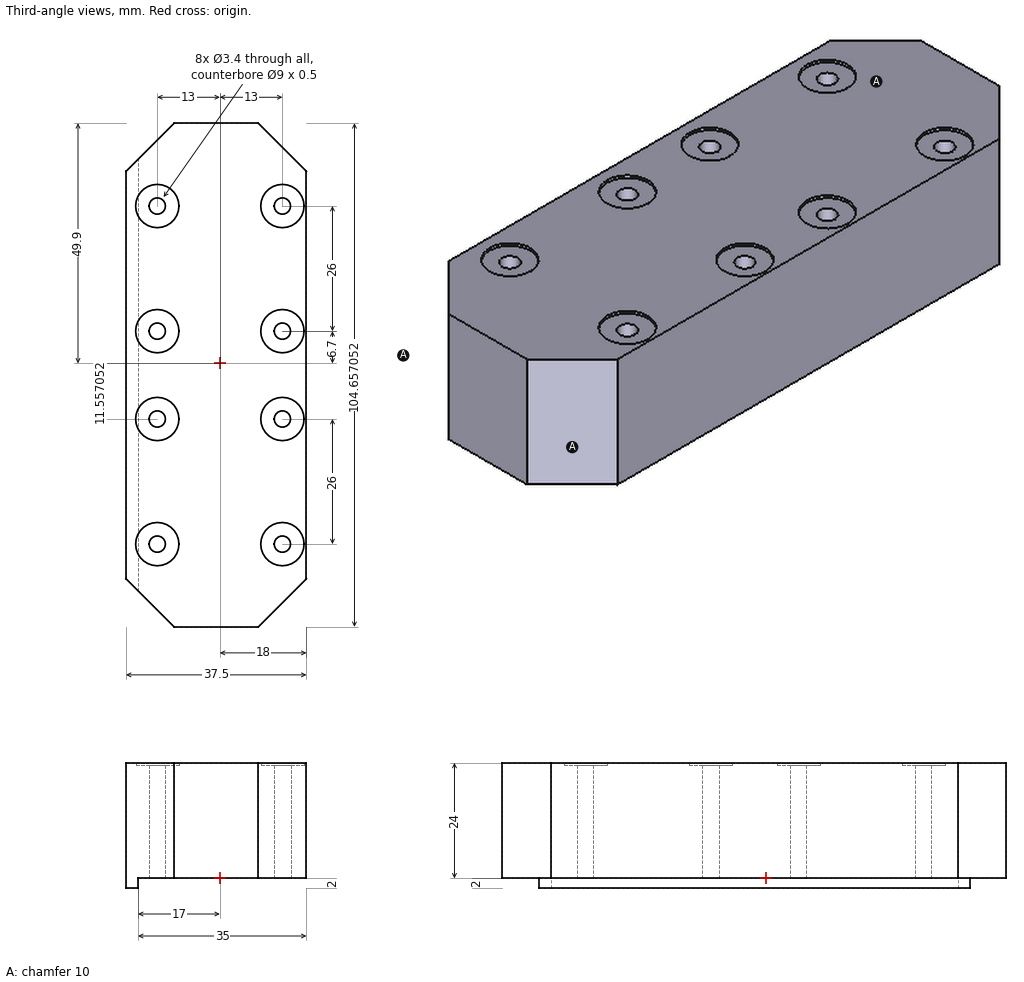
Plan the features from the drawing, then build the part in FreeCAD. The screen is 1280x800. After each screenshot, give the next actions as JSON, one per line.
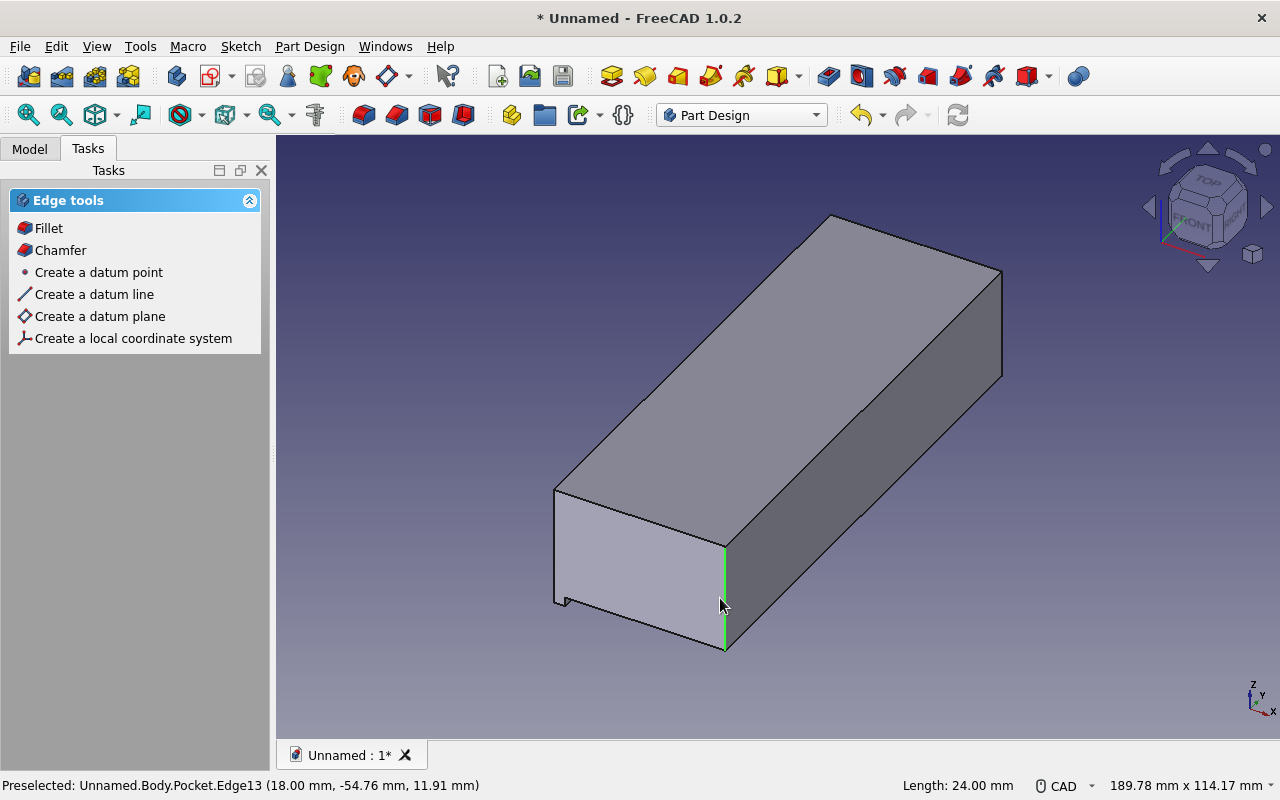
{"action": "key", "text": "0"}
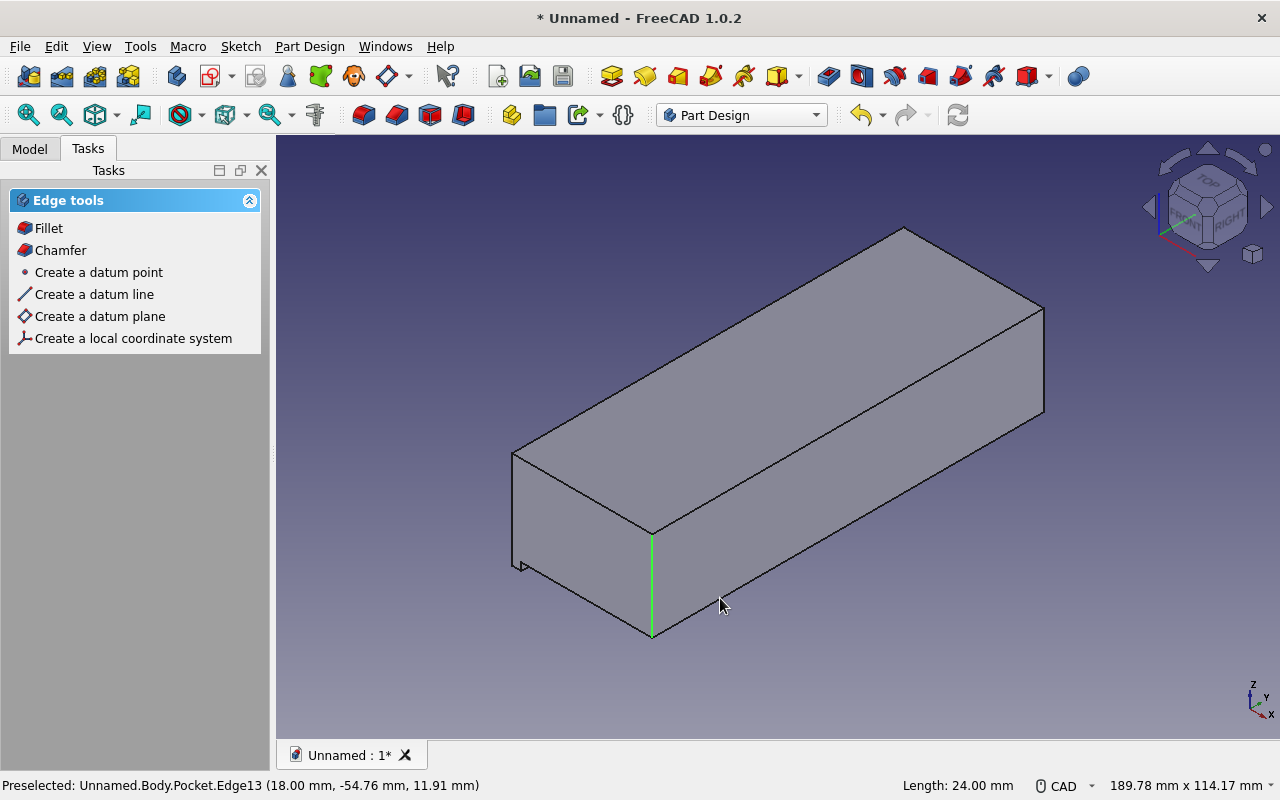
{"action": "key", "text": "2"}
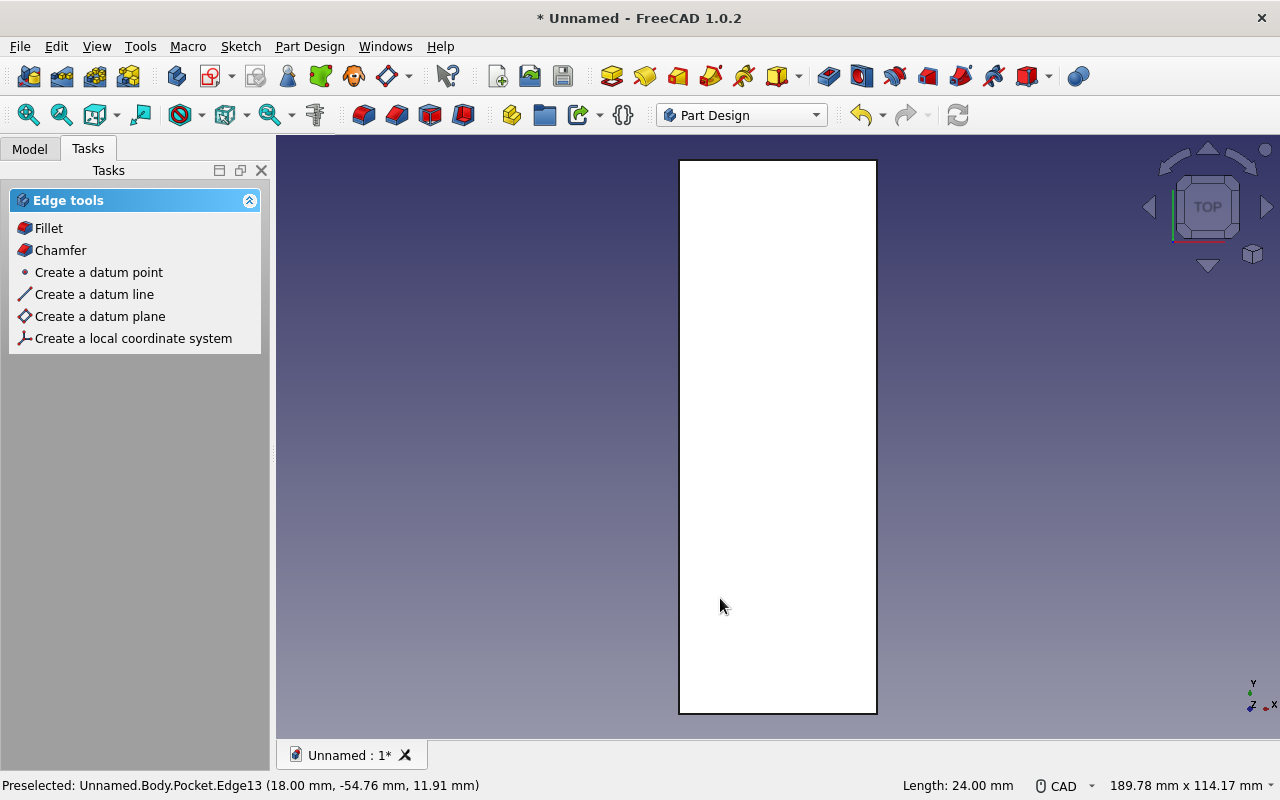
{"action": "key", "text": "1"}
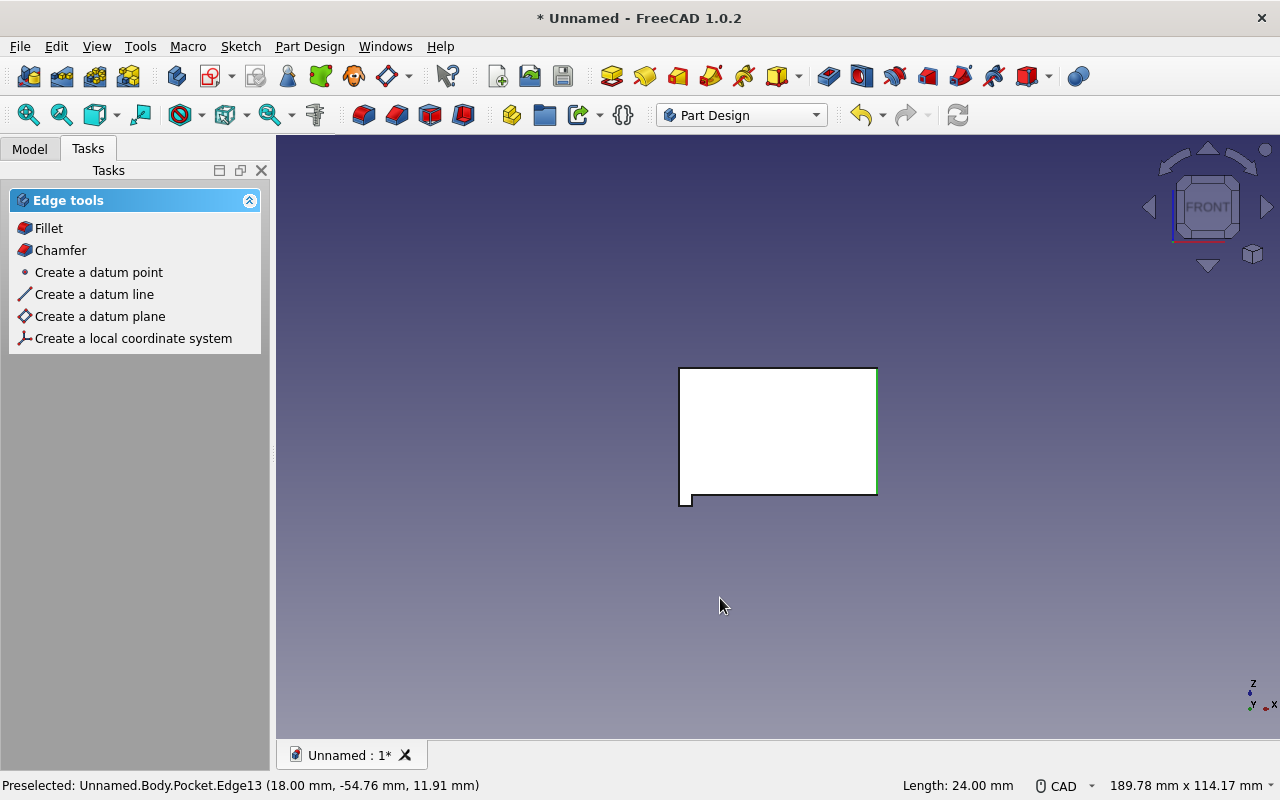
{"action": "left_click", "coordinate": [29, 116]}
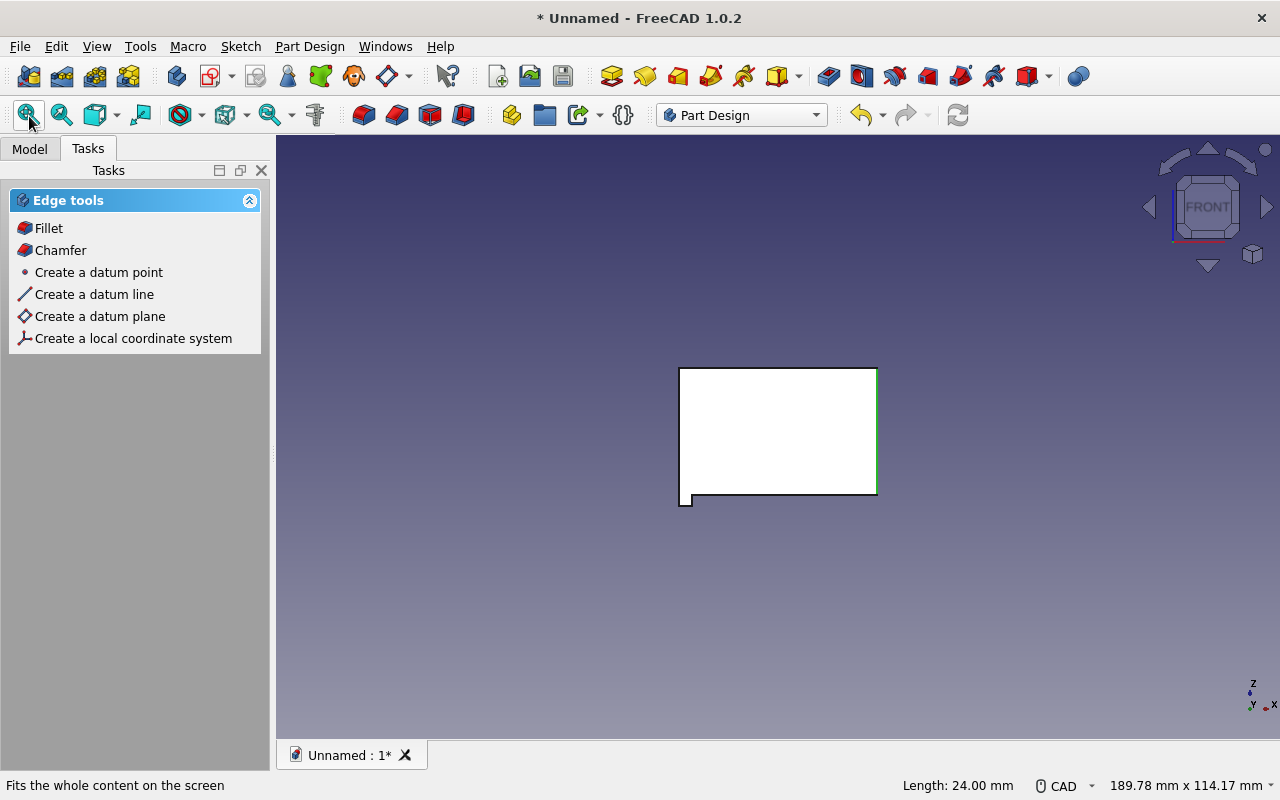
{"action": "left_click", "coordinate": [679, 436], "text": "ctrl"}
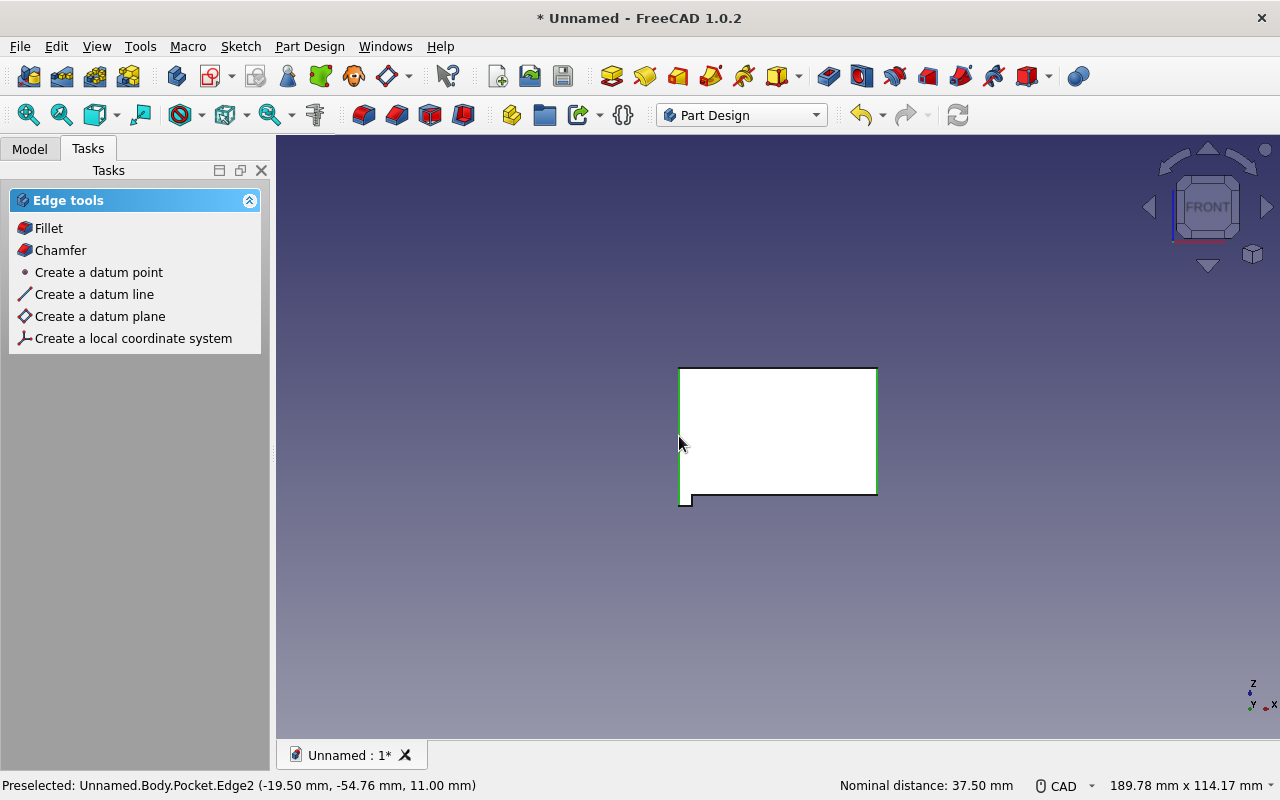
{"action": "key", "text": "3"}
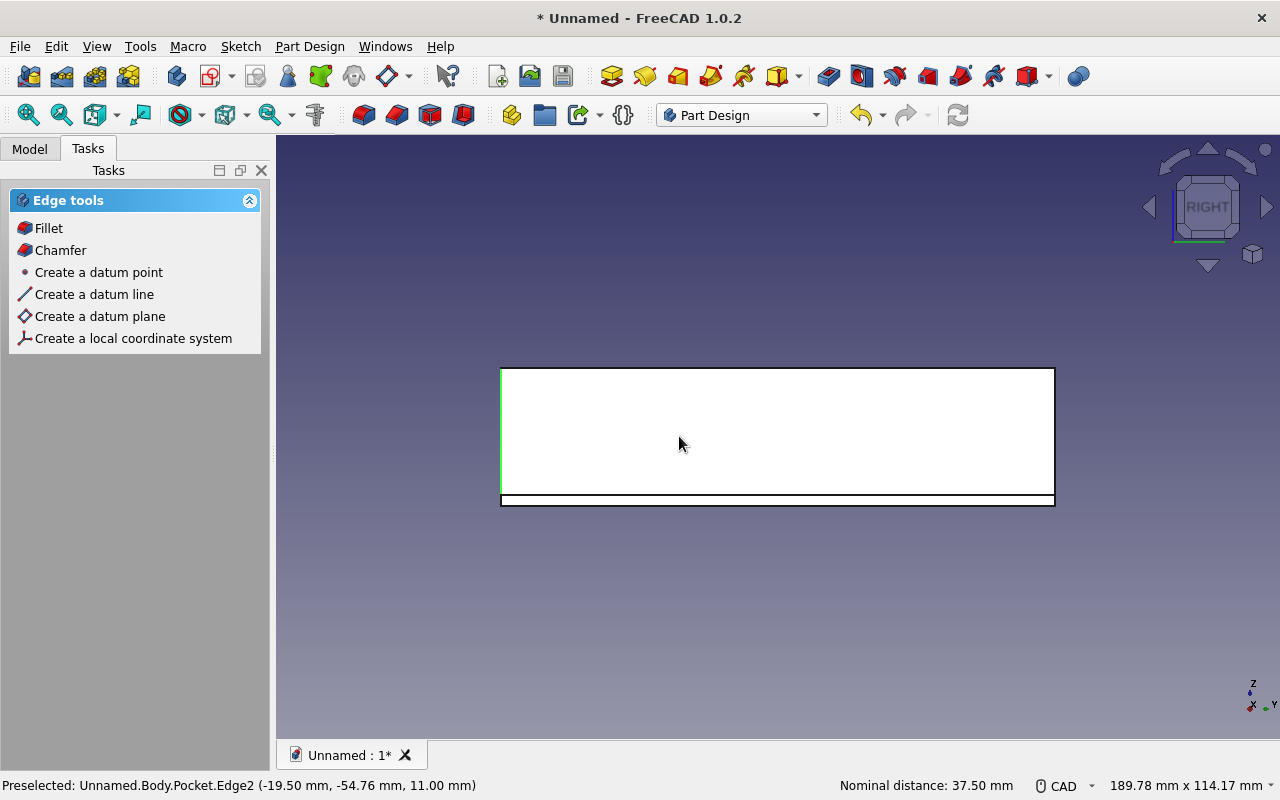
{"action": "left_click", "coordinate": [1055, 431], "text": "ctrl"}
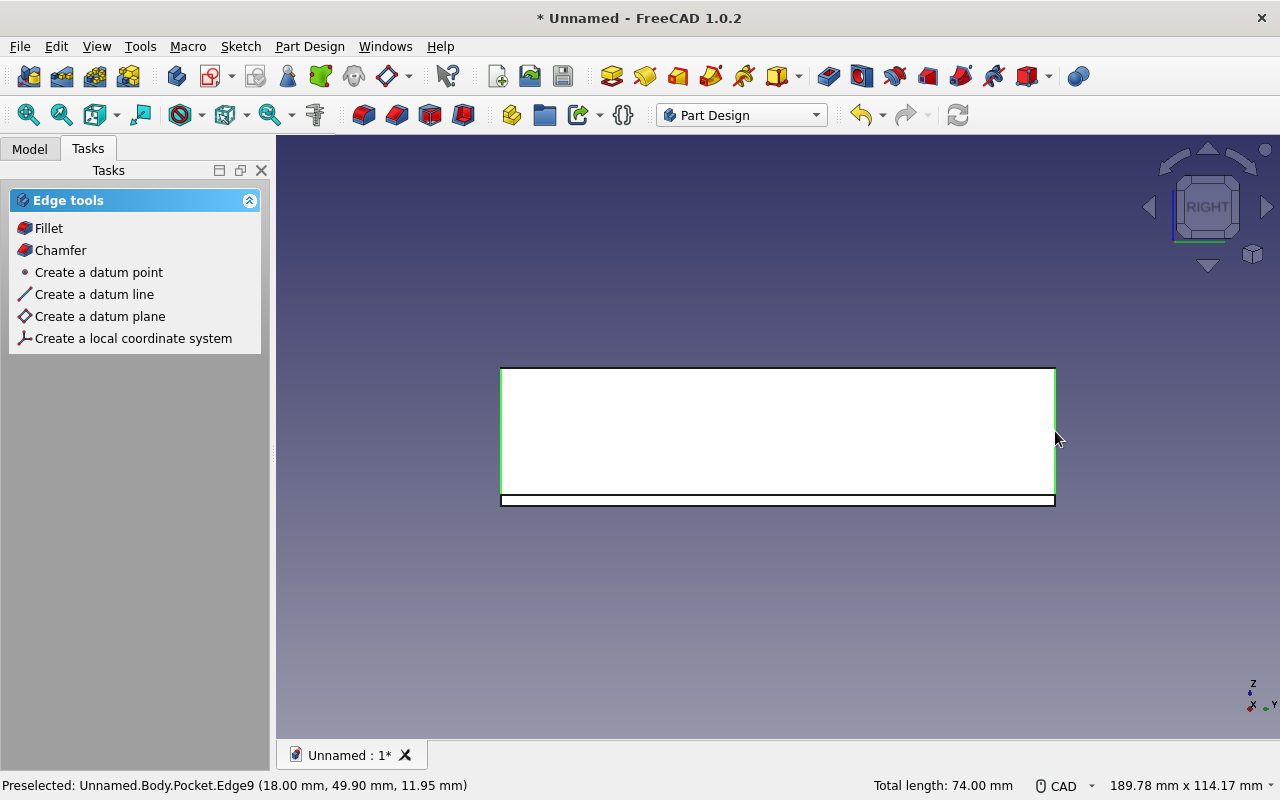
{"action": "key", "text": "5"}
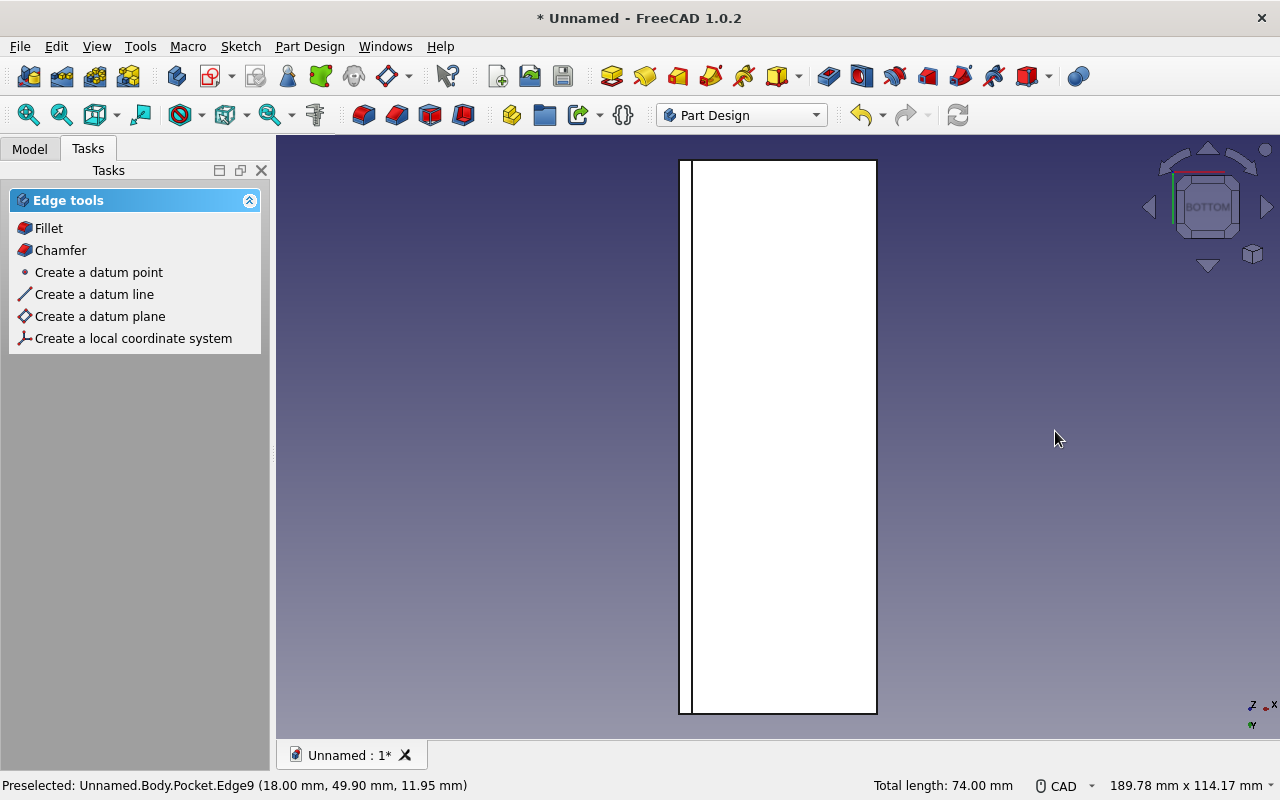
{"action": "key", "text": "4"}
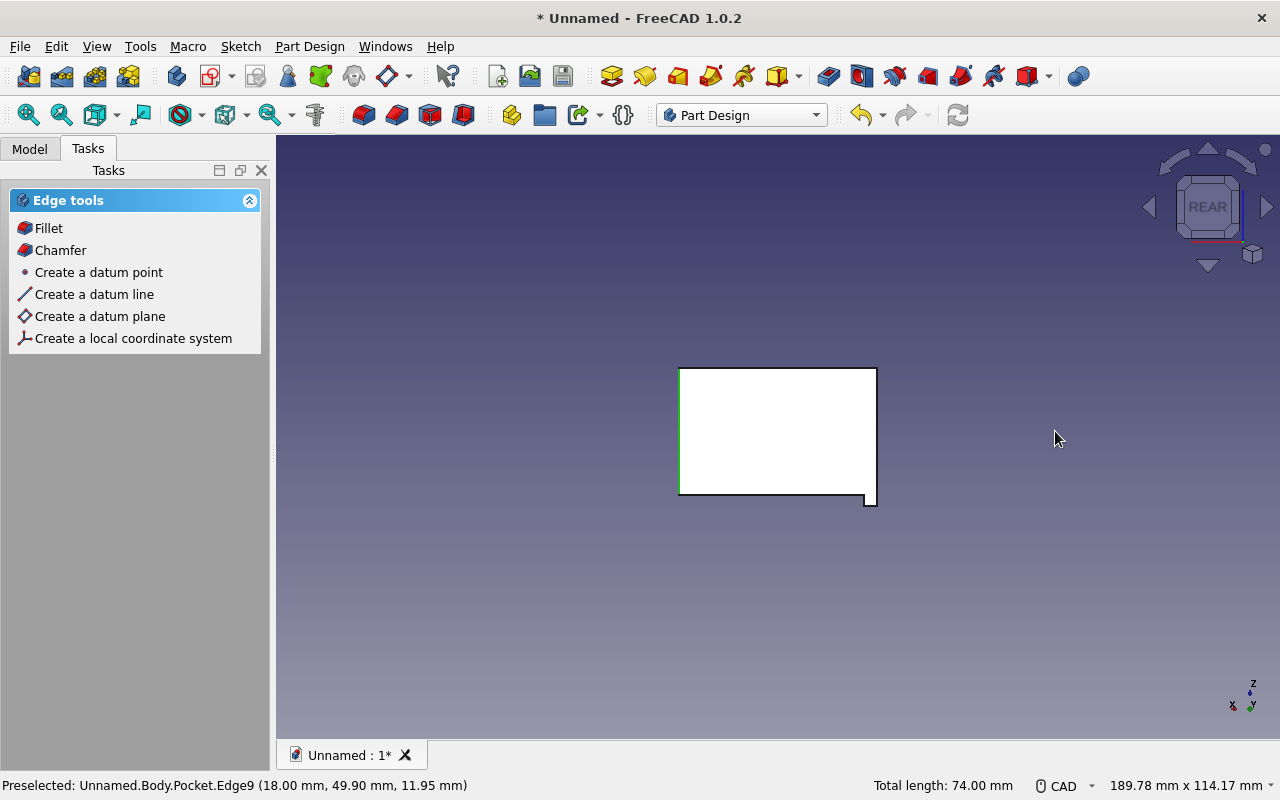
{"action": "left_click", "coordinate": [29, 116]}